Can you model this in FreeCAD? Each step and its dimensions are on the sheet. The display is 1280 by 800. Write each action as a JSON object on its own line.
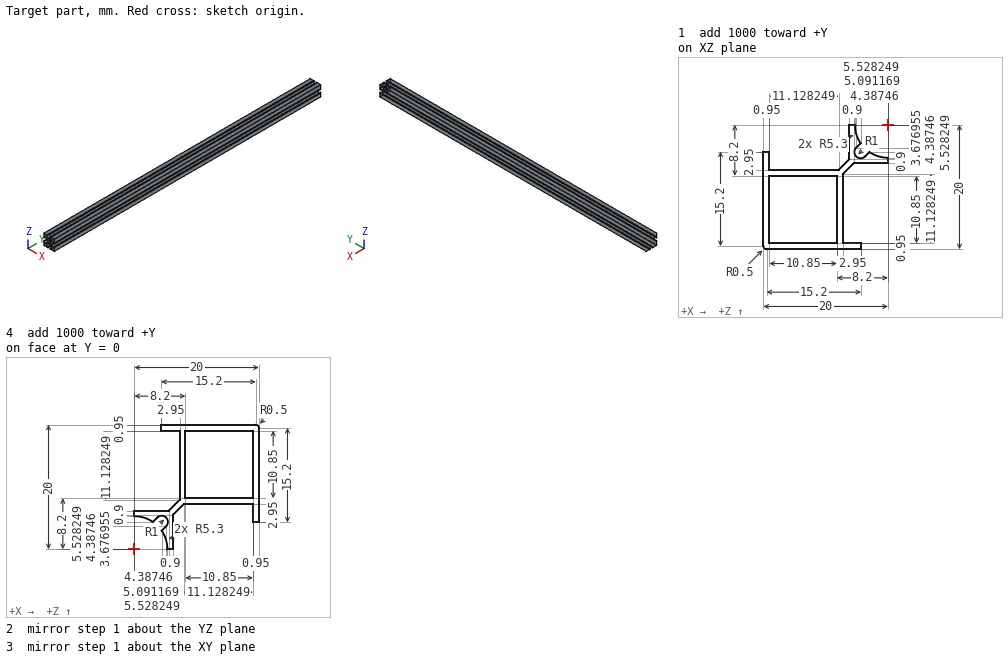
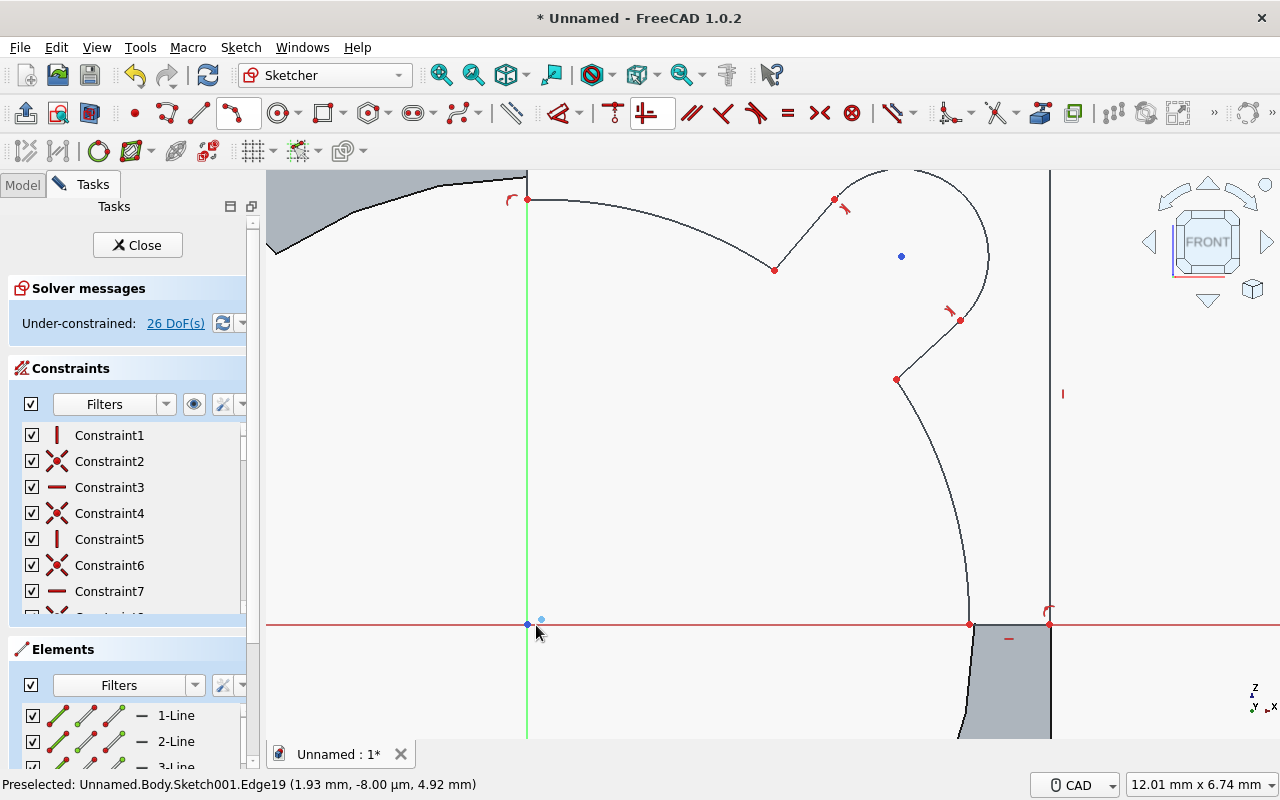
{"action": "left_click_drag", "start_coordinate": [517, 609], "coordinate": [551, 635]}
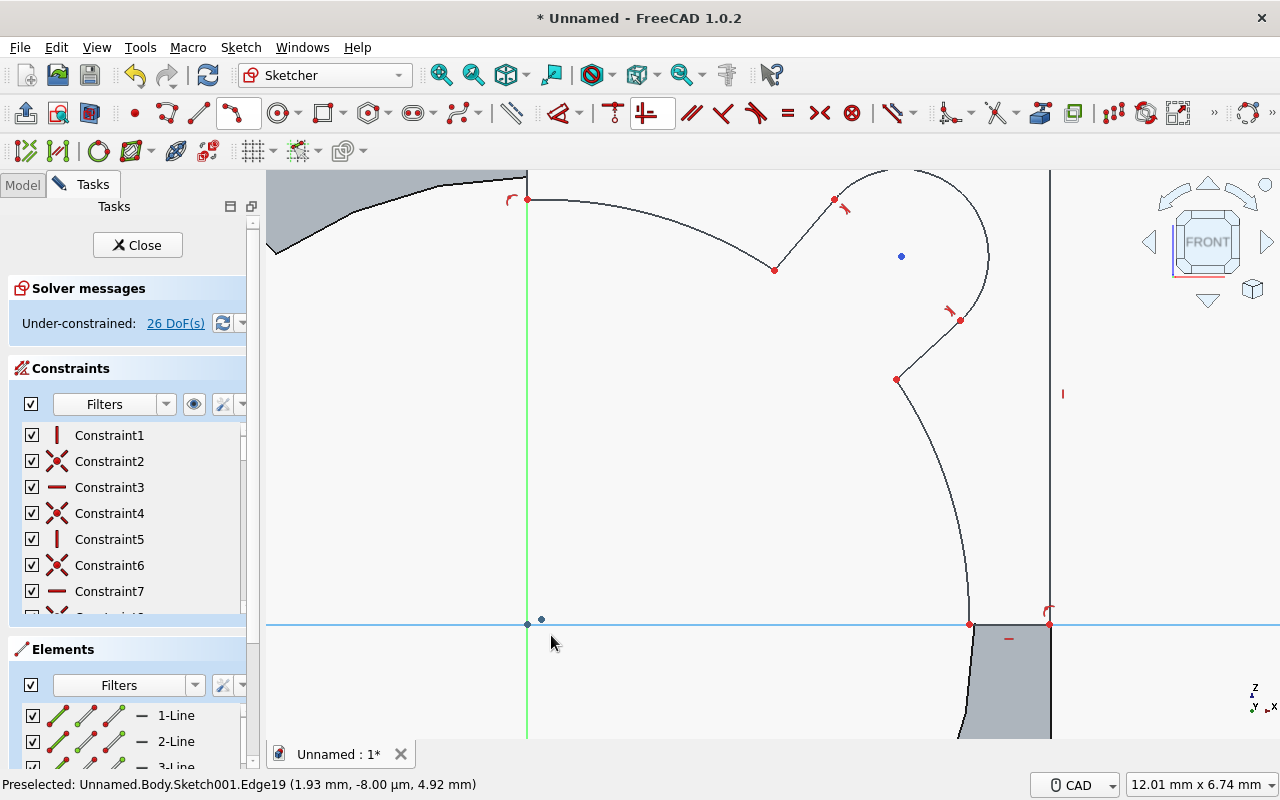
{"action": "left_click", "coordinate": [614, 114]}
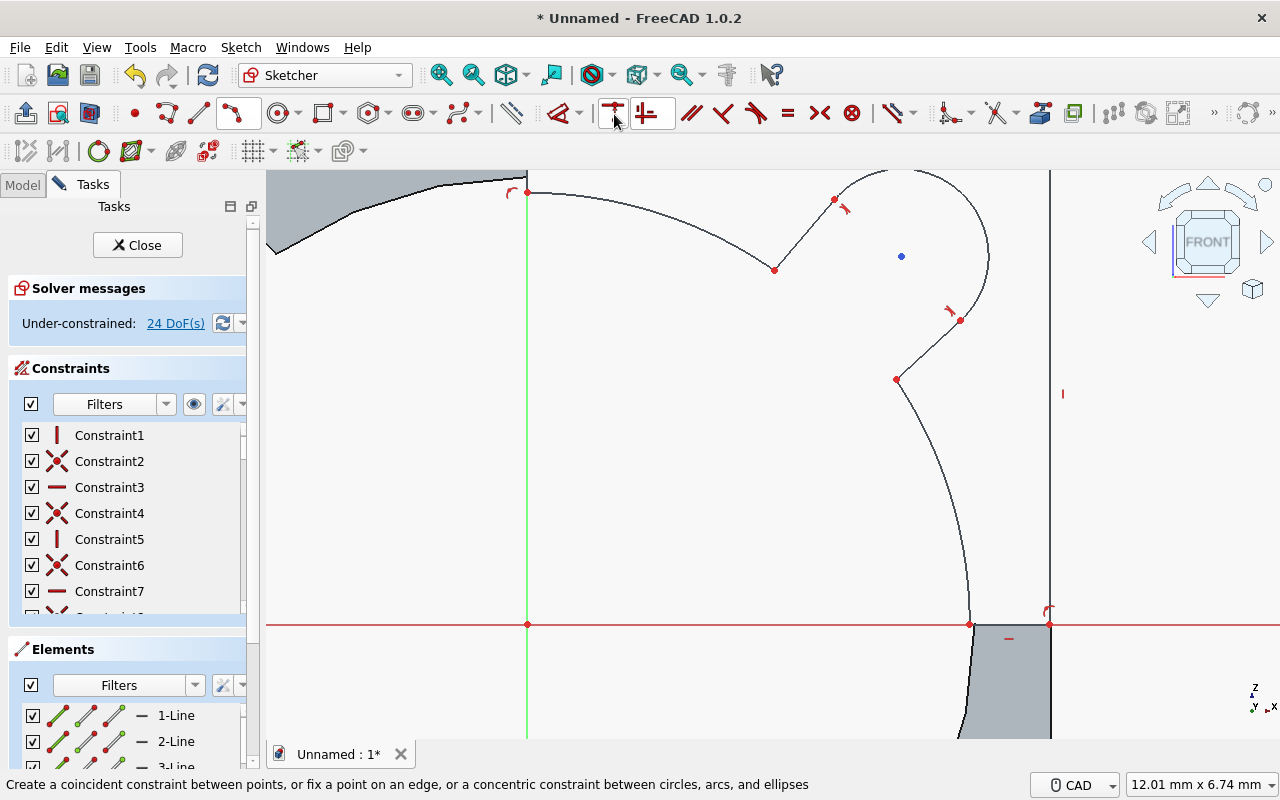
{"action": "scroll", "coordinate": [536, 625], "scroll_direction": "down", "scroll_amount": 8}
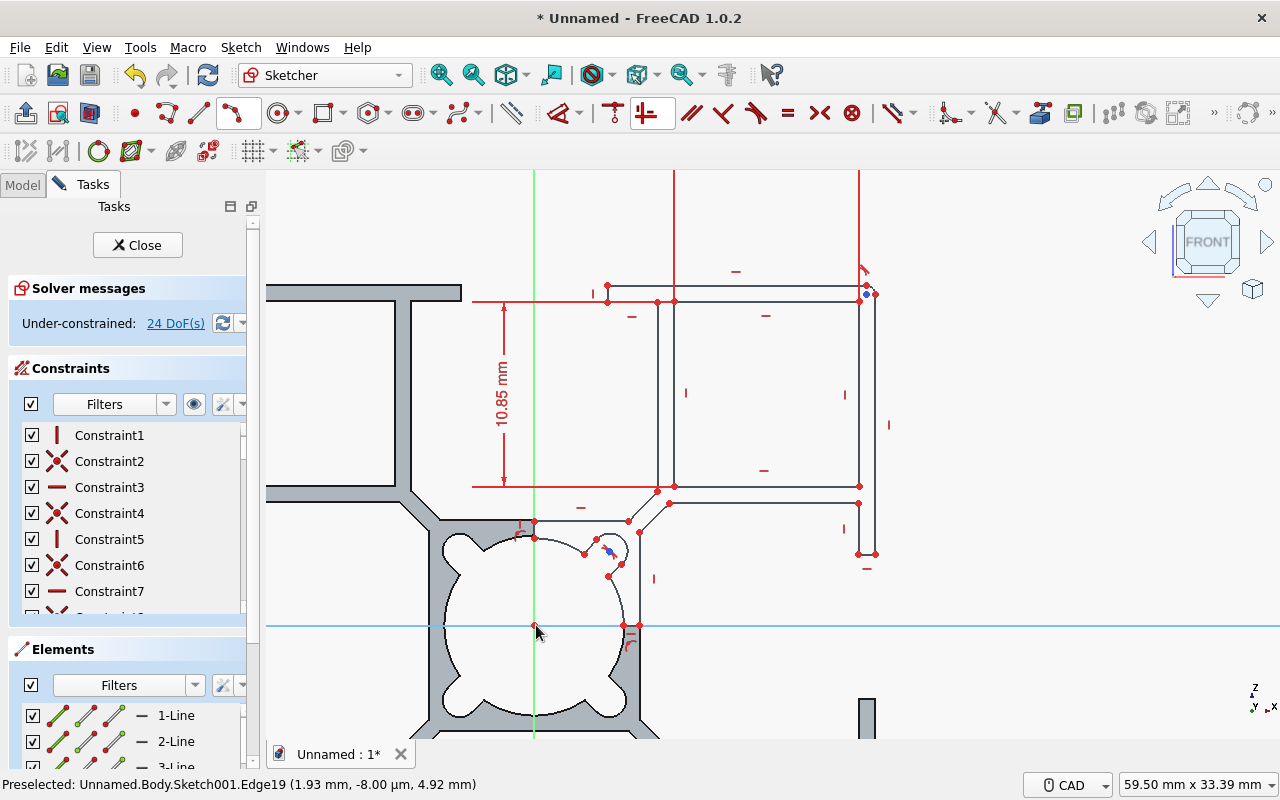
{"action": "left_click", "coordinate": [622, 610]}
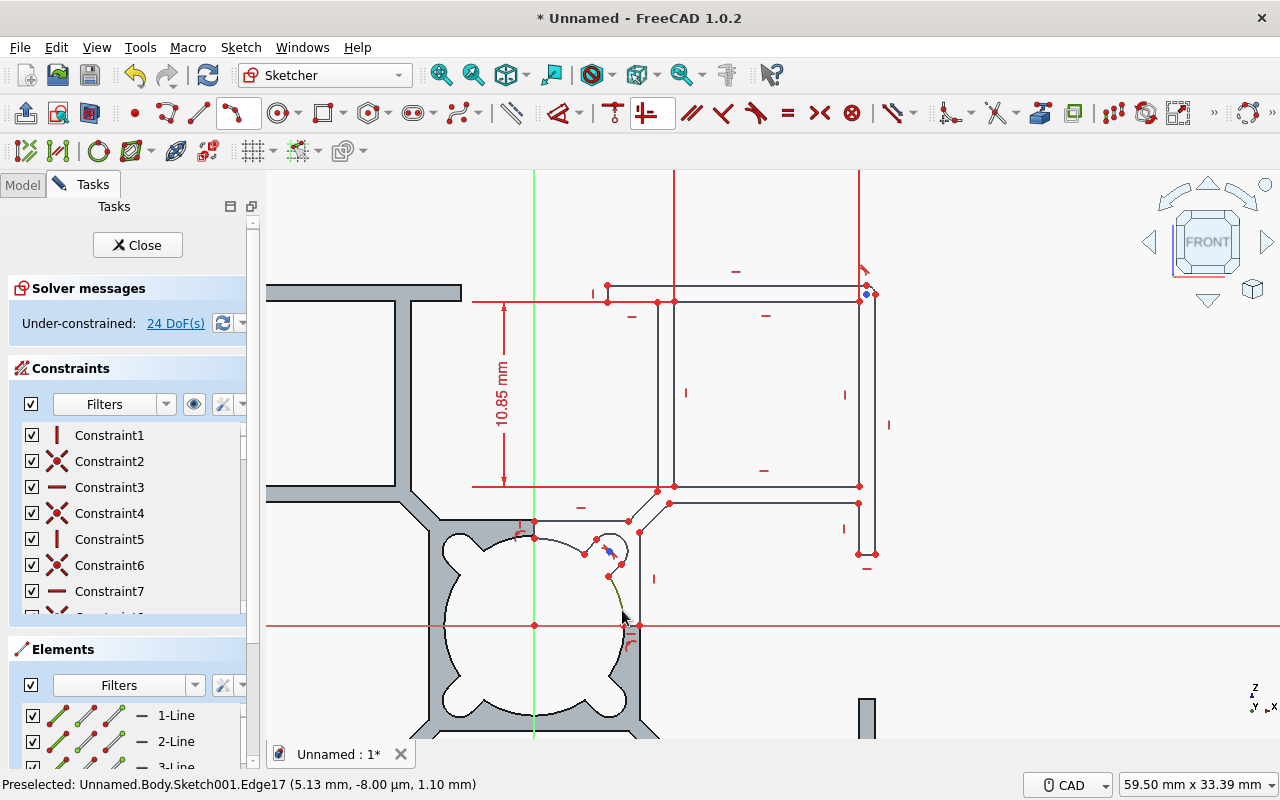
{"action": "left_click", "coordinate": [571, 546]}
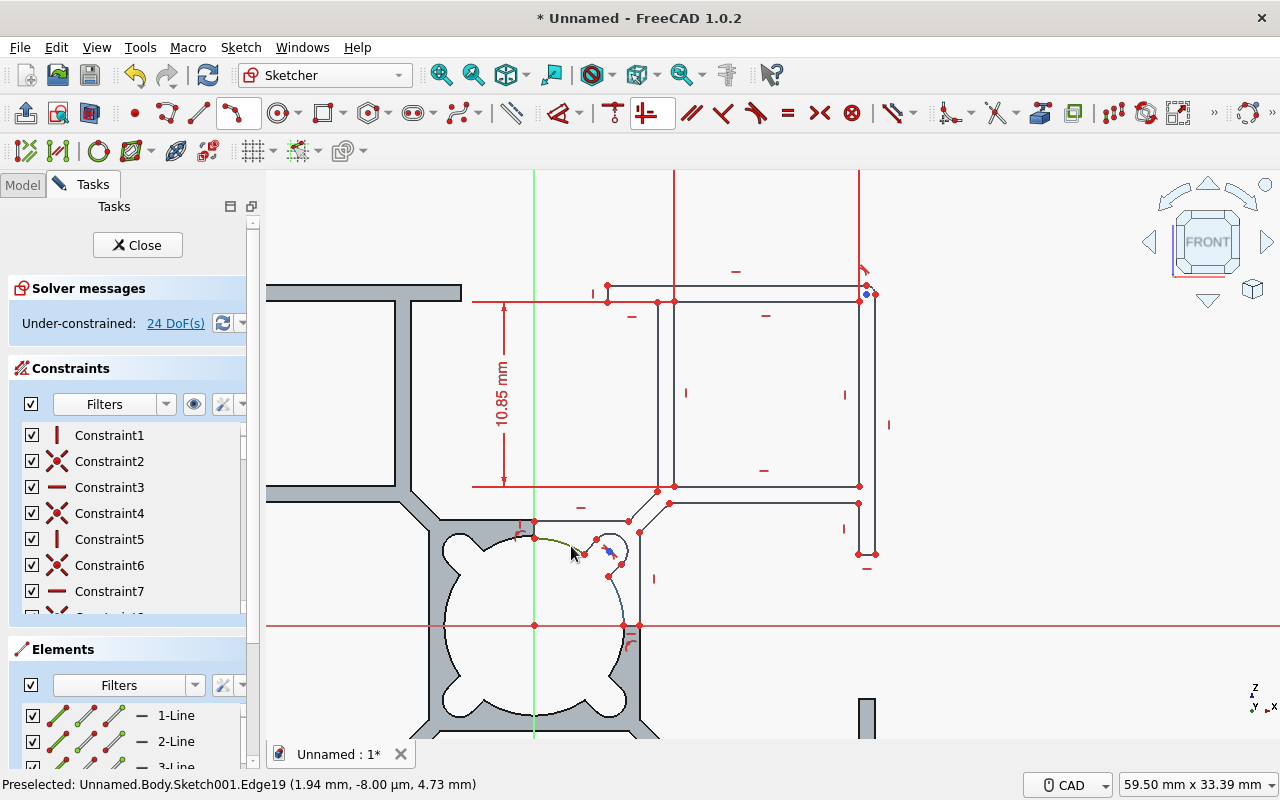
{"action": "left_click", "coordinate": [788, 114]}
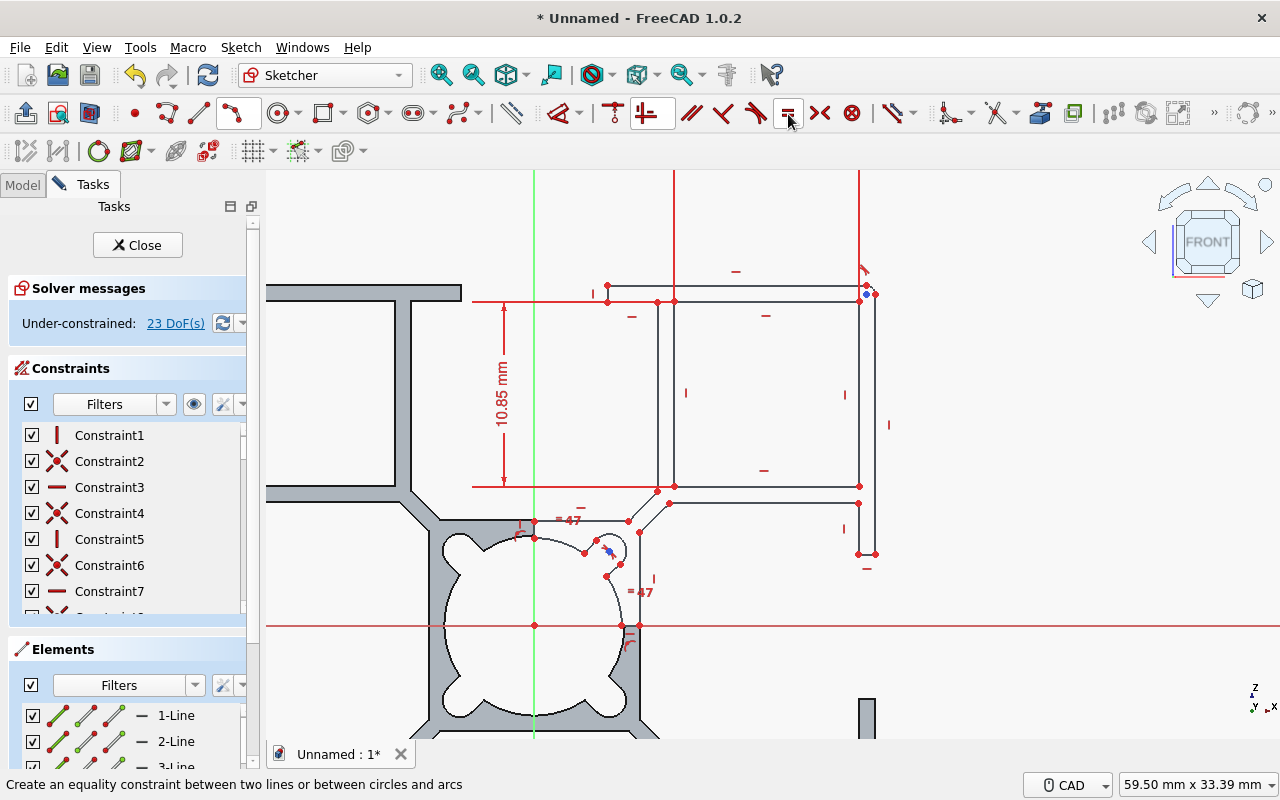
{"action": "left_click", "coordinate": [558, 114]}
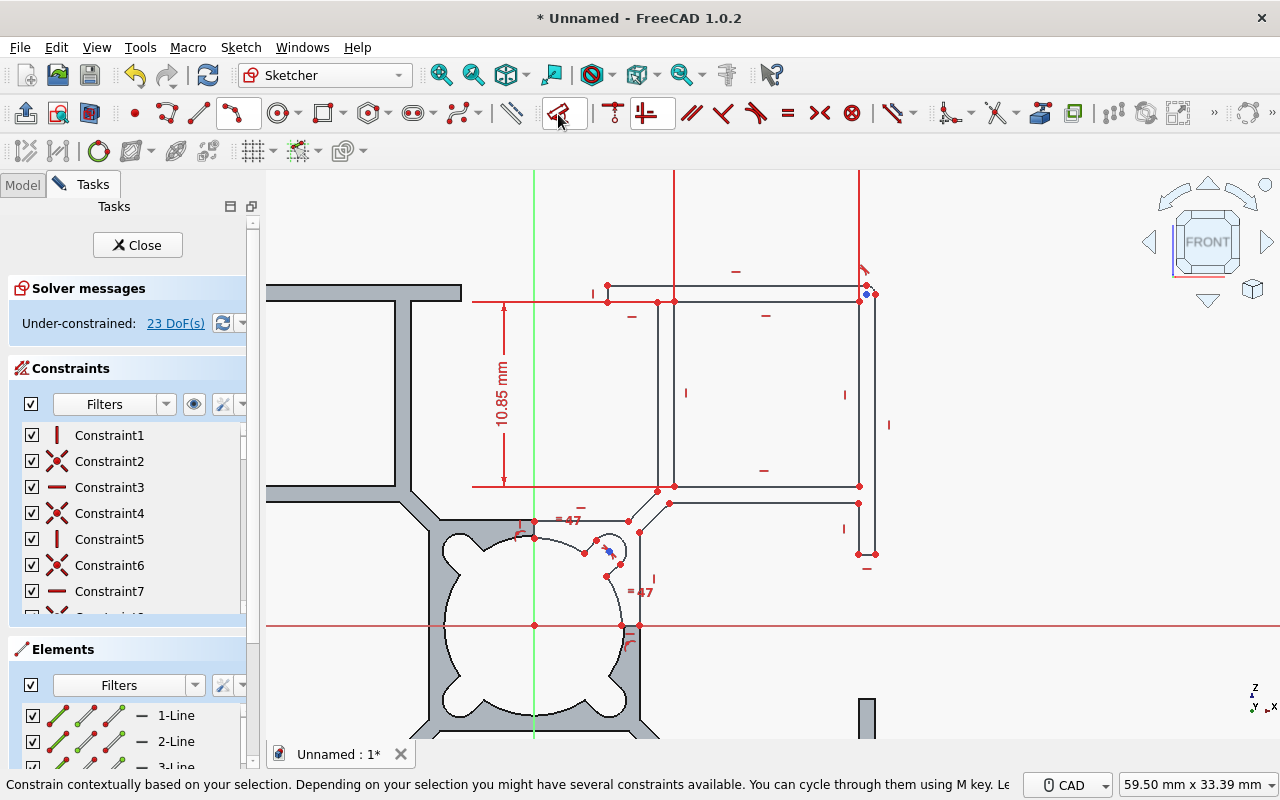
{"action": "left_click", "coordinate": [620, 610]}
{"action": "left_click", "coordinate": [647, 663]}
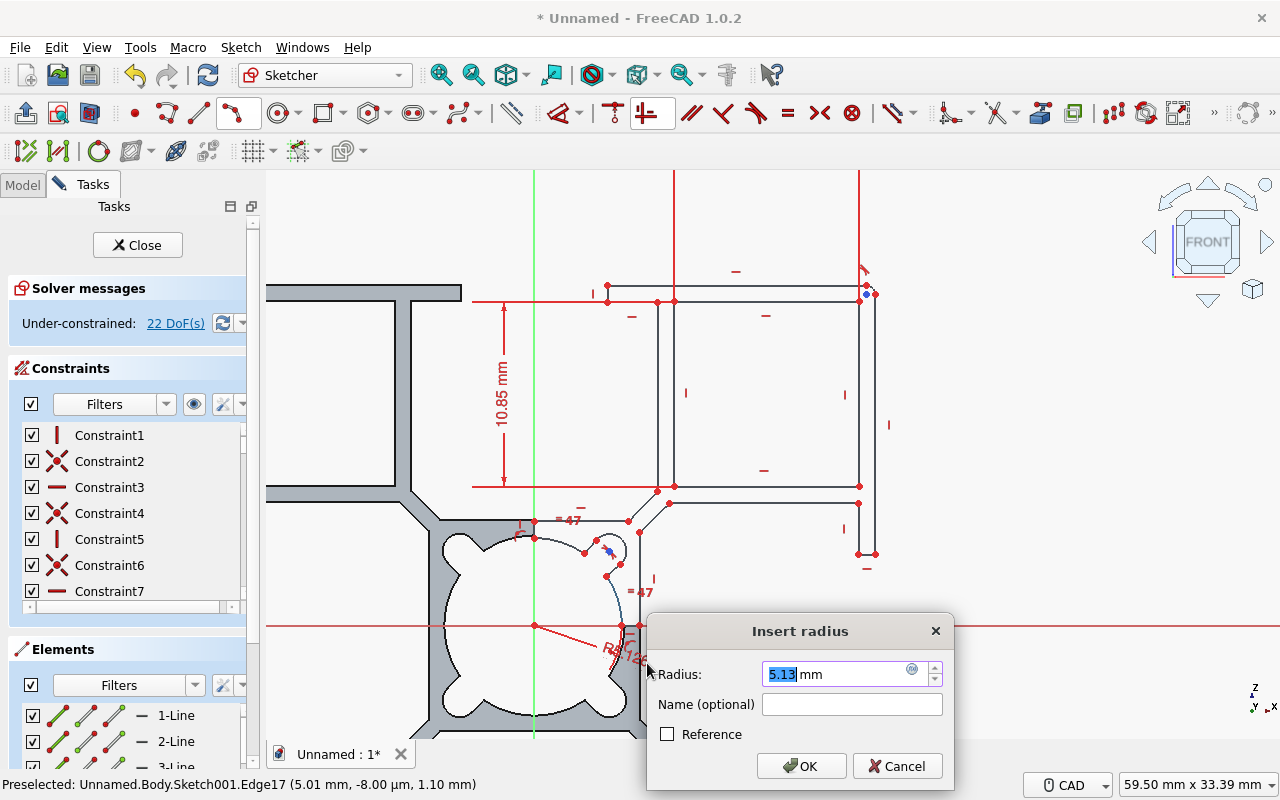
{"action": "type", "text": "5.3"}
{"action": "key", "text": "Return"}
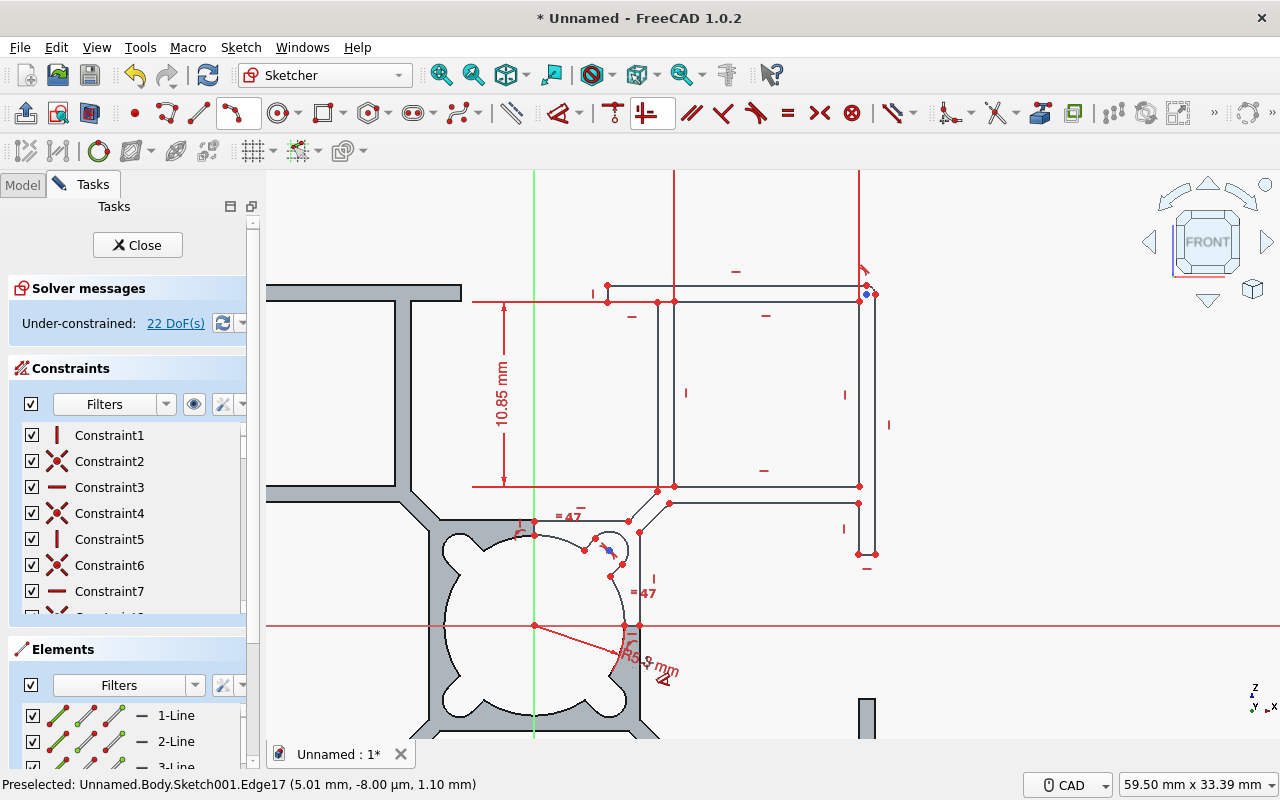
{"action": "scroll", "coordinate": [628, 547], "scroll_direction": "up", "scroll_amount": 5}